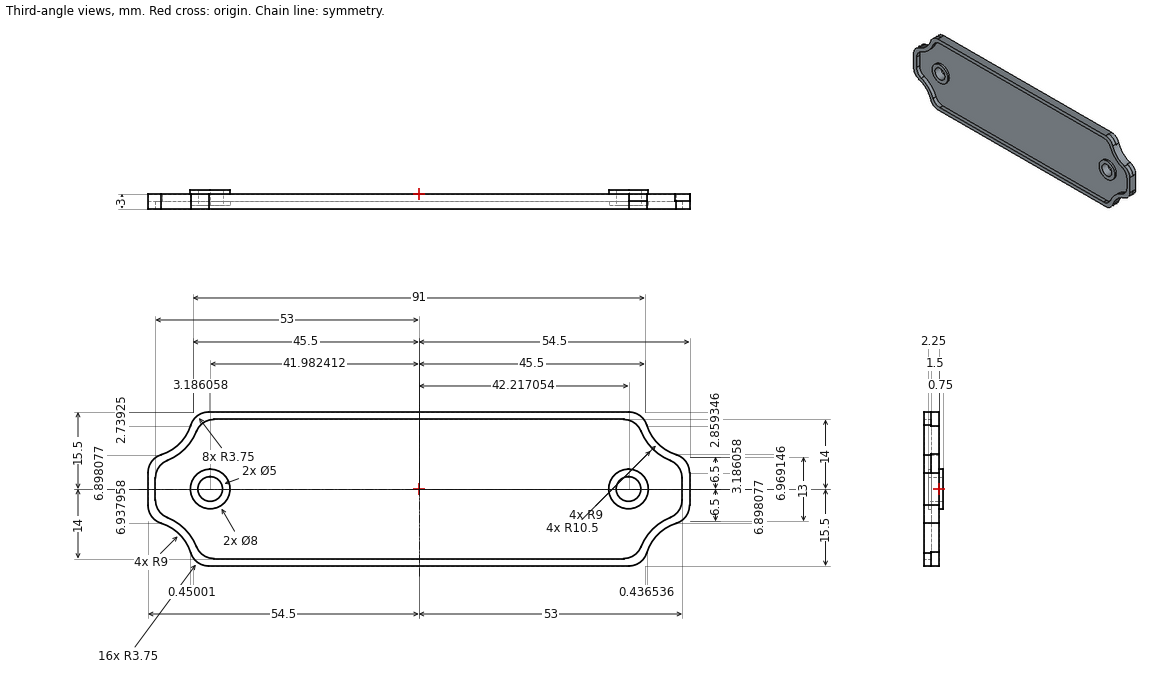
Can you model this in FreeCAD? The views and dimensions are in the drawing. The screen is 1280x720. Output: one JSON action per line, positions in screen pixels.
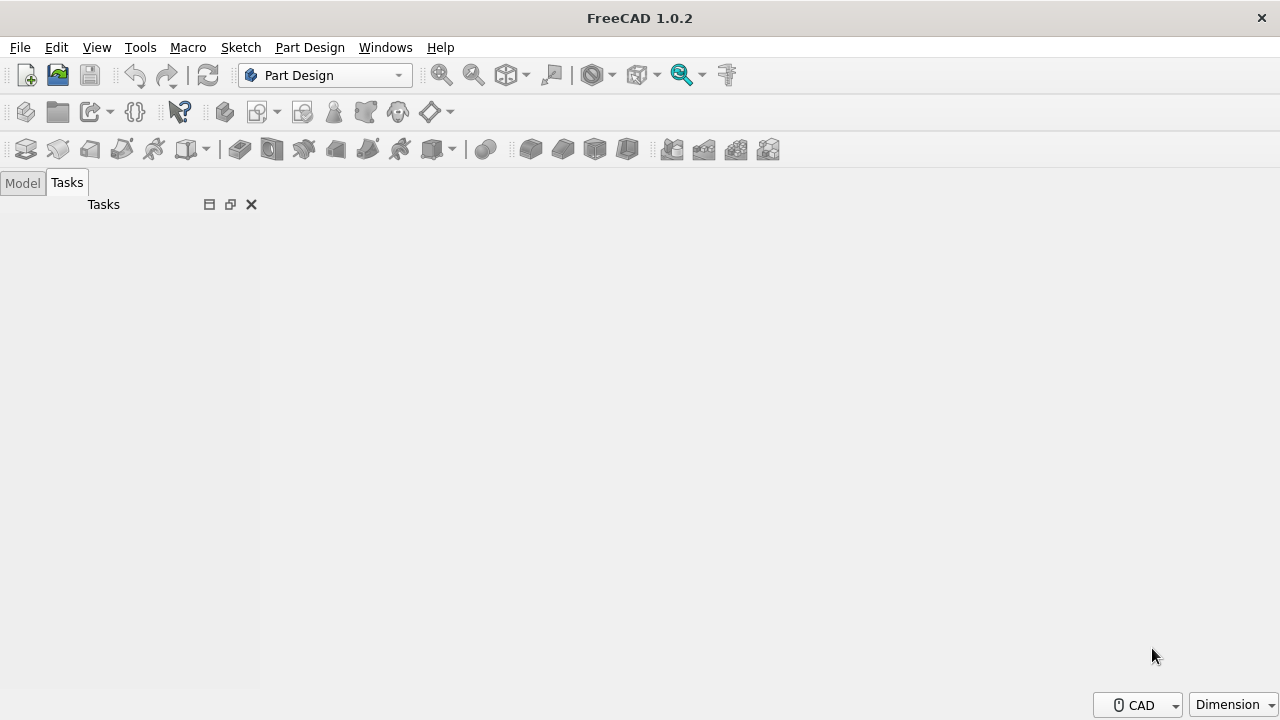
{"action": "left_click", "coordinate": [26, 76]}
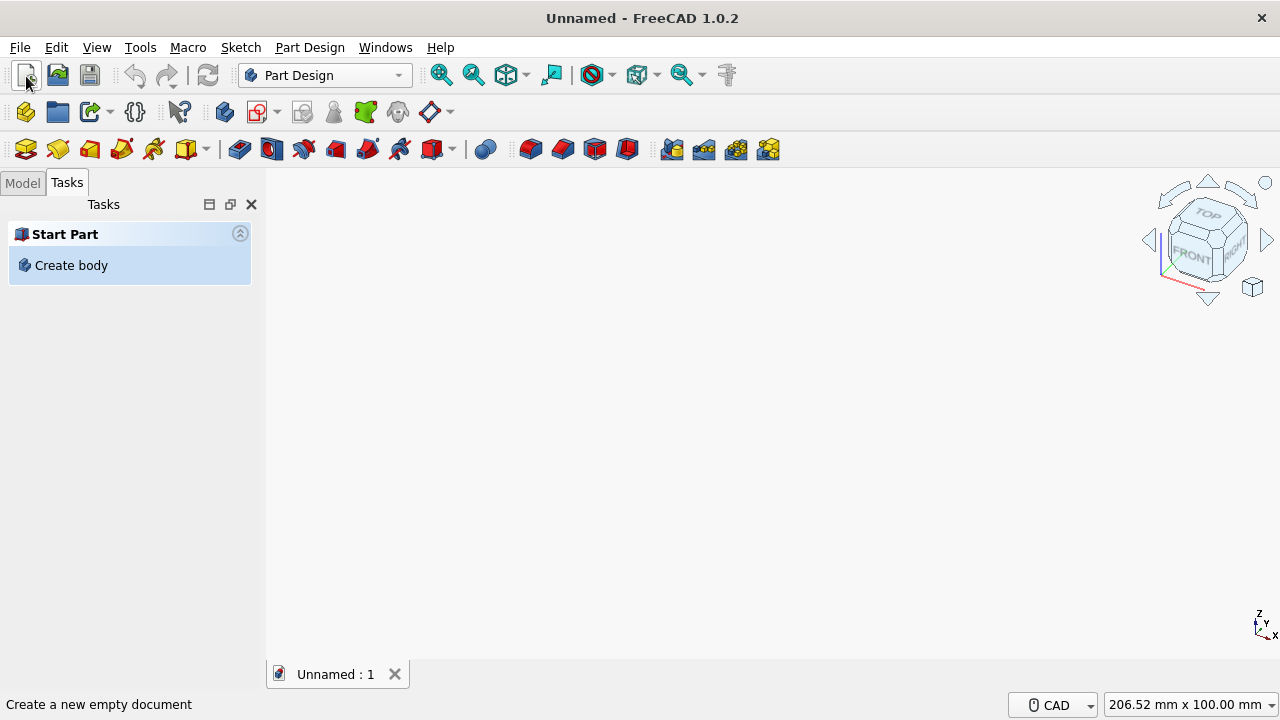
{"action": "left_click", "coordinate": [258, 112]}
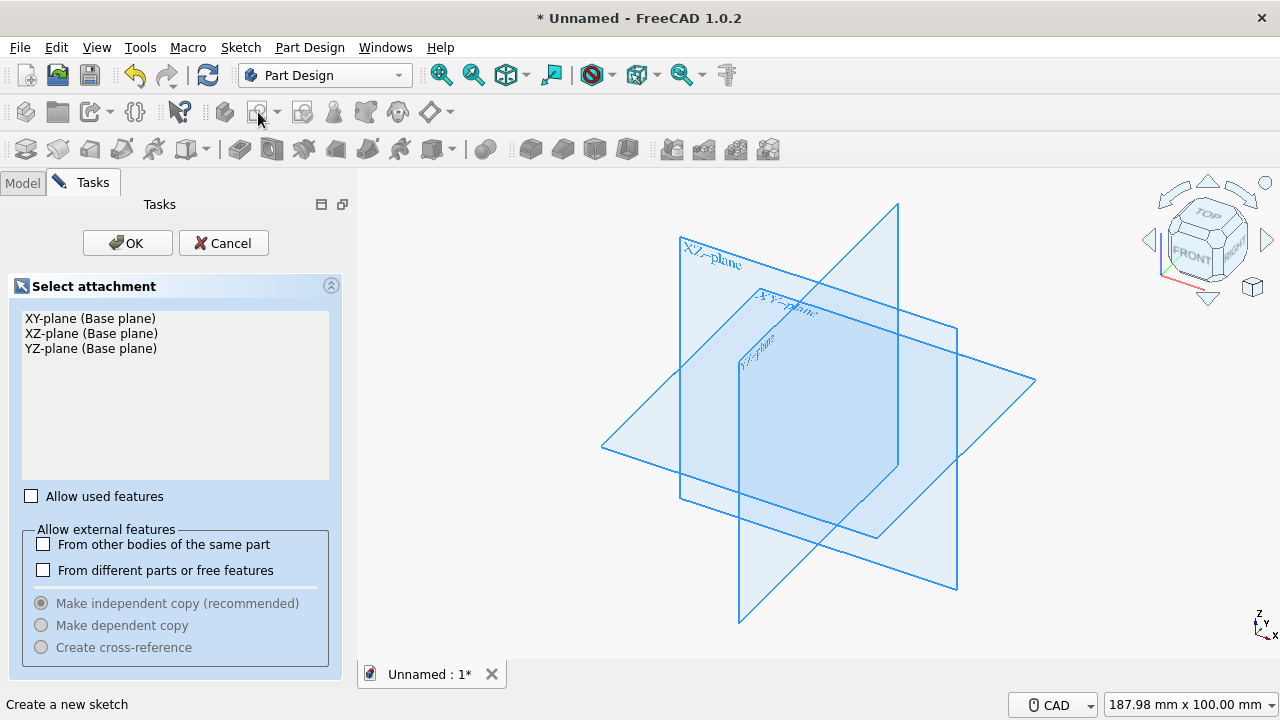
{"action": "left_click", "coordinate": [82, 334]}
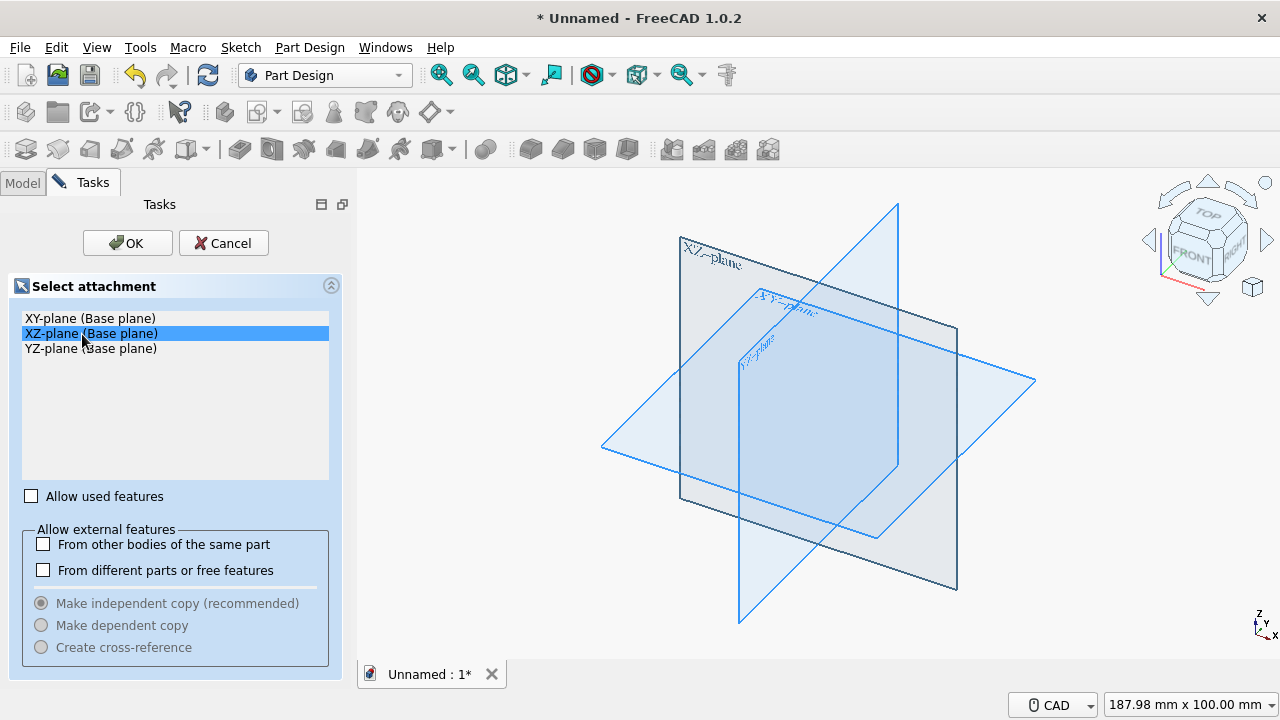
{"action": "left_click", "coordinate": [128, 243]}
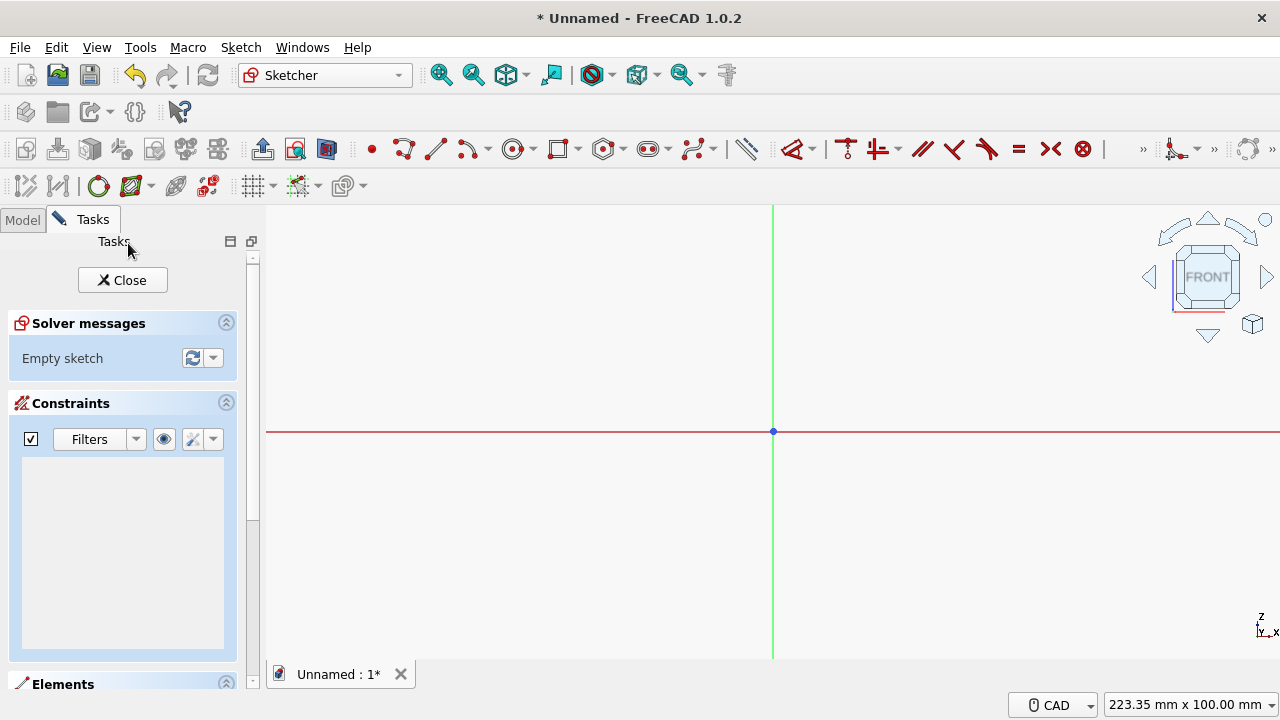
{"action": "left_click", "coordinate": [436, 150]}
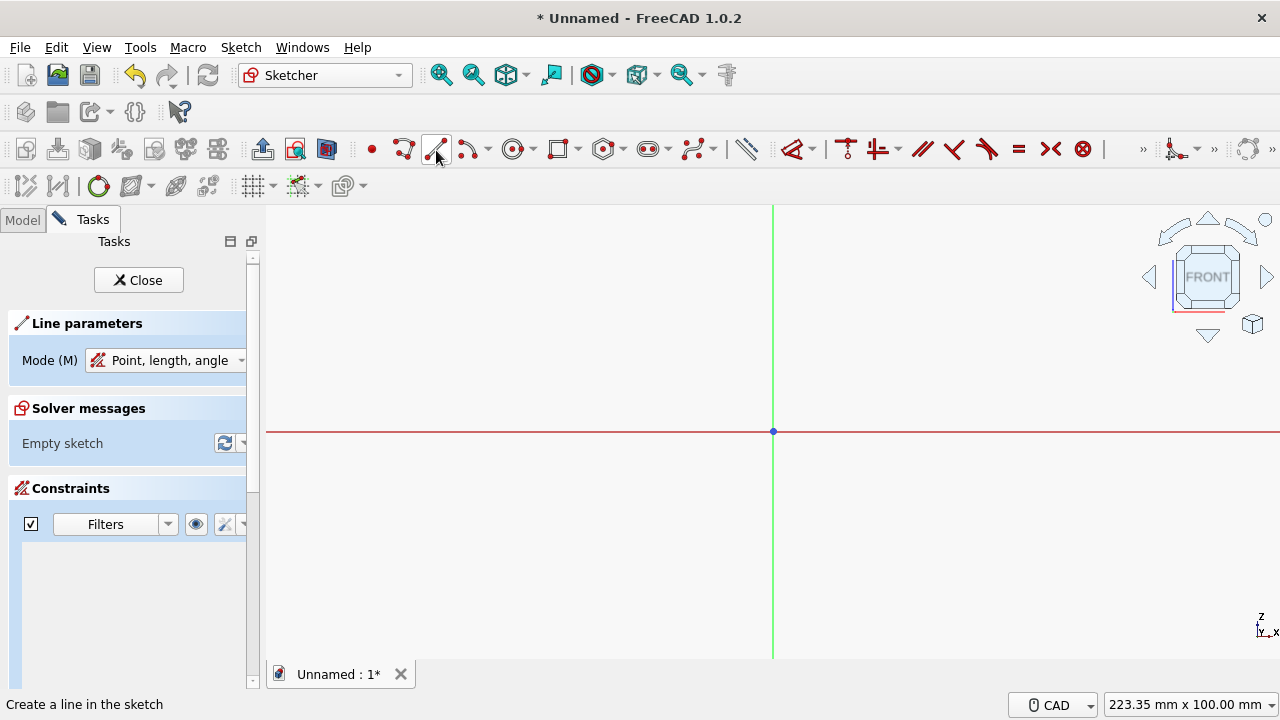
{"action": "left_click", "coordinate": [566, 362]}
{"action": "left_click", "coordinate": [980, 362]}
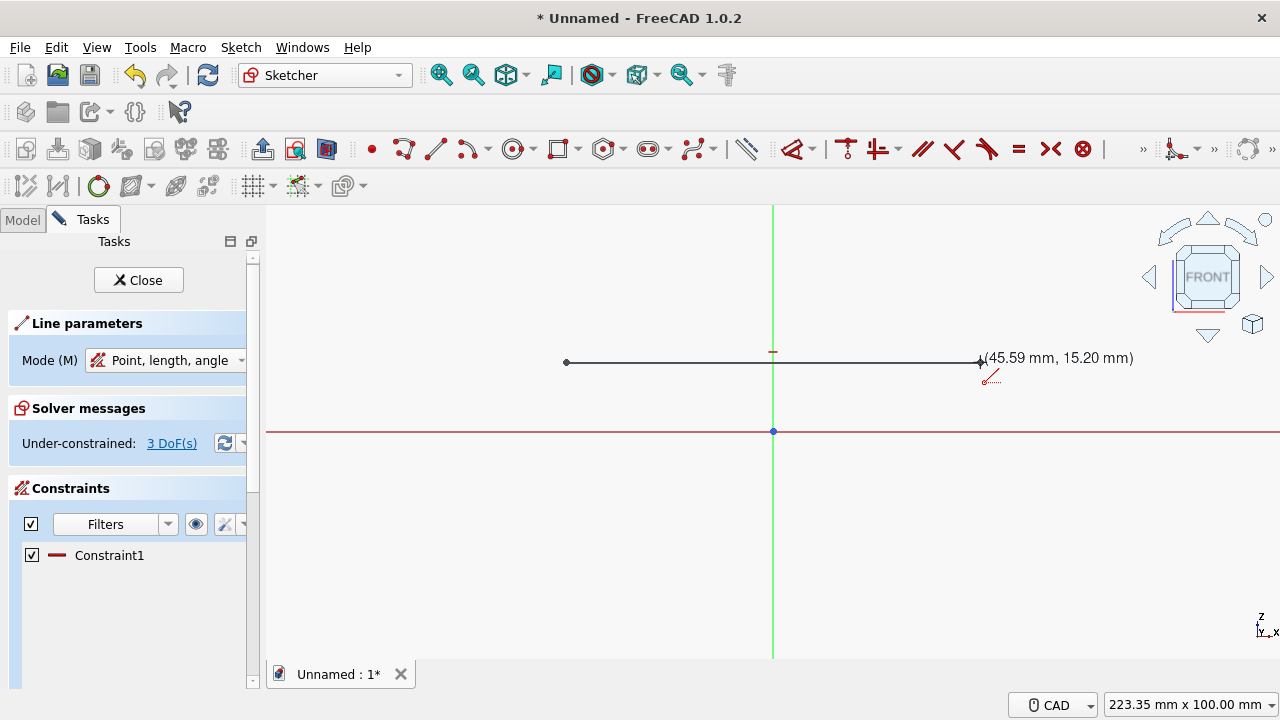
{"action": "left_click", "coordinate": [1020, 402]}
{"action": "left_click", "coordinate": [1020, 462]}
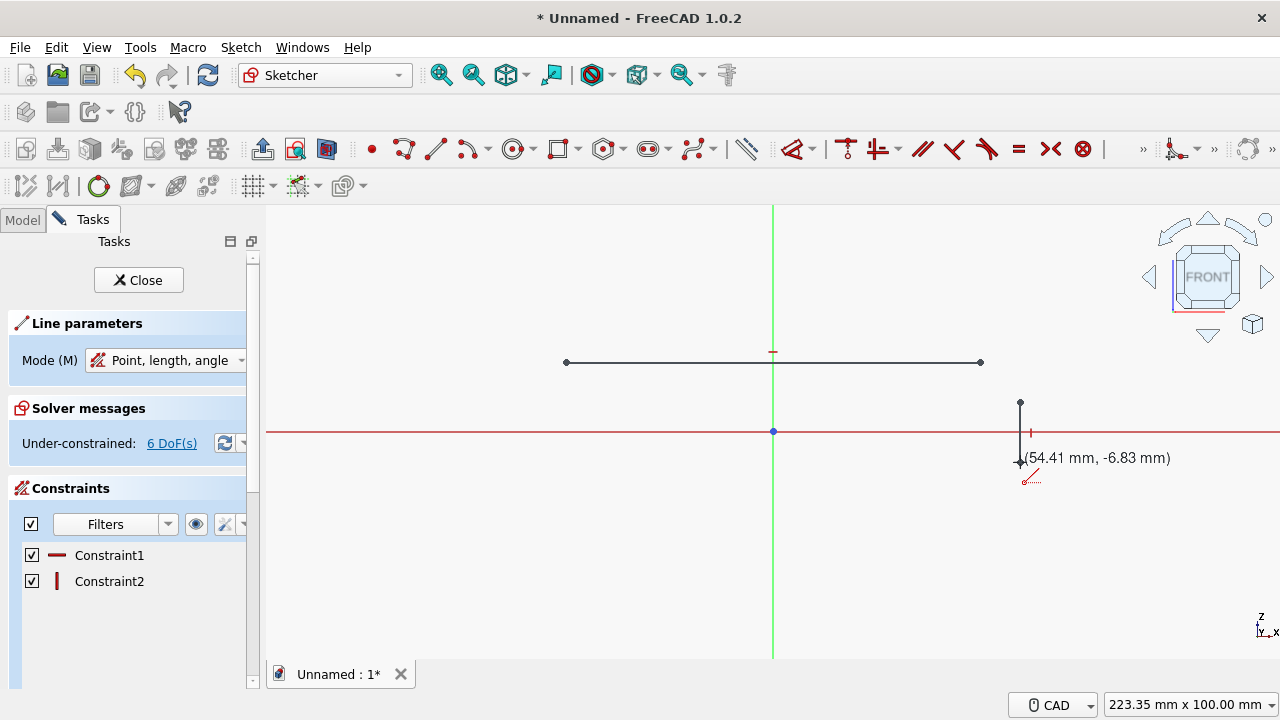
{"action": "left_click", "coordinate": [980, 502]}
{"action": "left_click", "coordinate": [566, 502]}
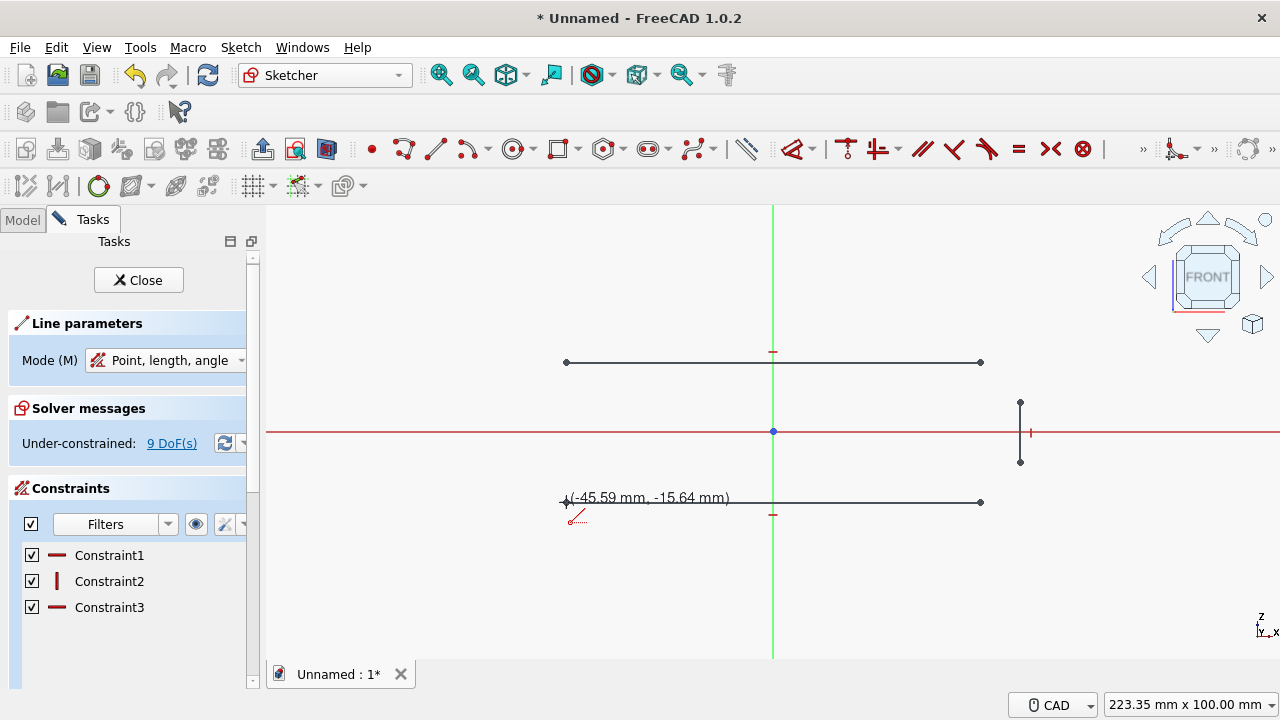
{"action": "left_click", "coordinate": [526, 462]}
{"action": "left_click", "coordinate": [526, 402]}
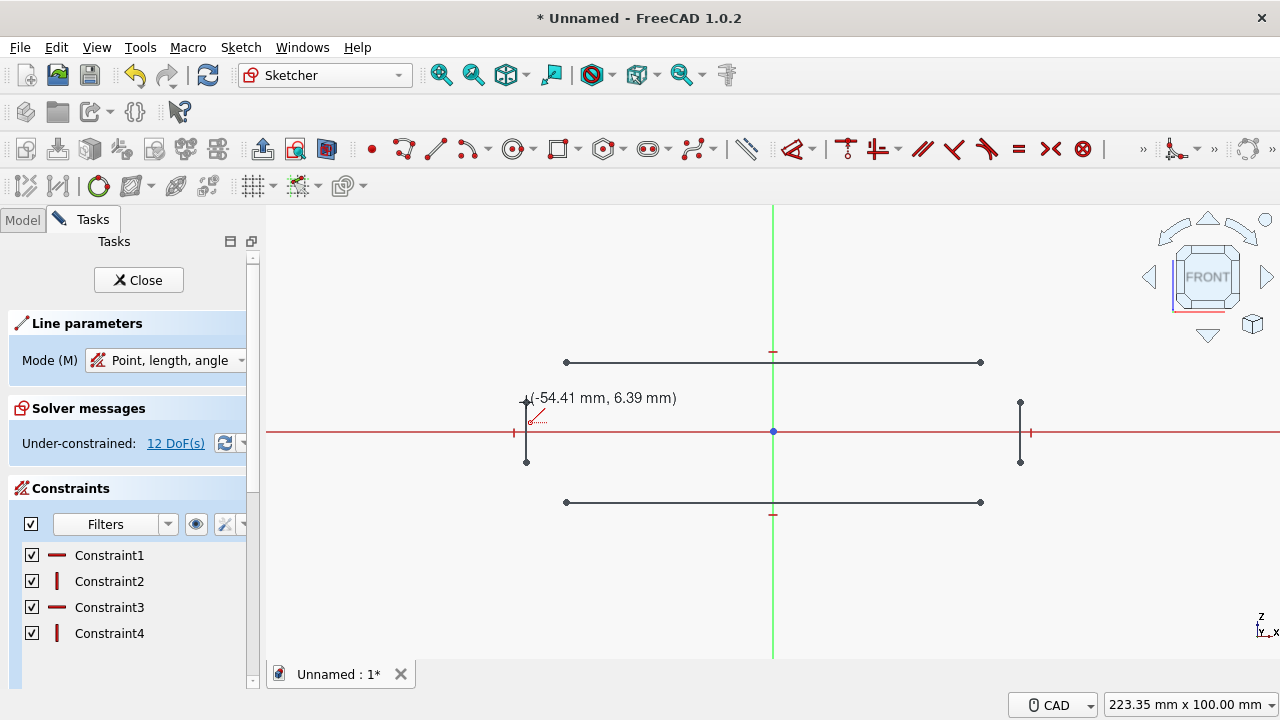
{"action": "key", "text": "g 3 a"}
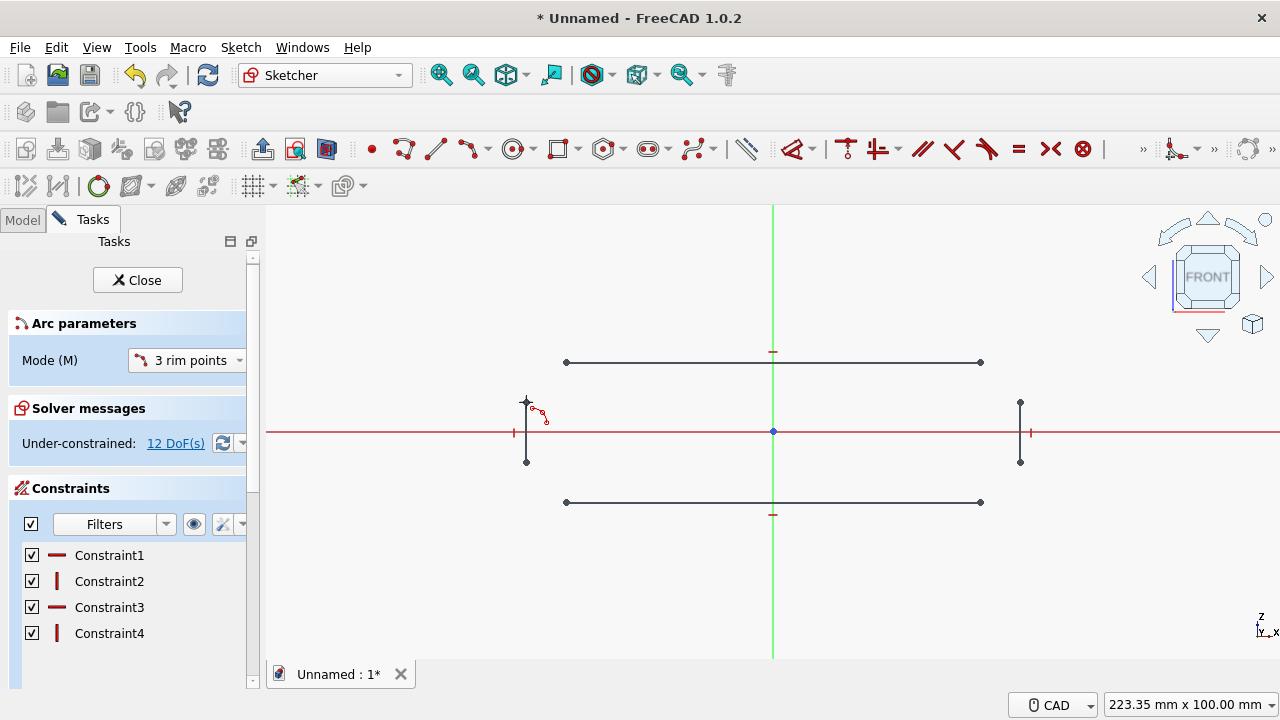
{"action": "left_click", "coordinate": [980, 363]}
{"action": "left_click", "coordinate": [1020, 403]}